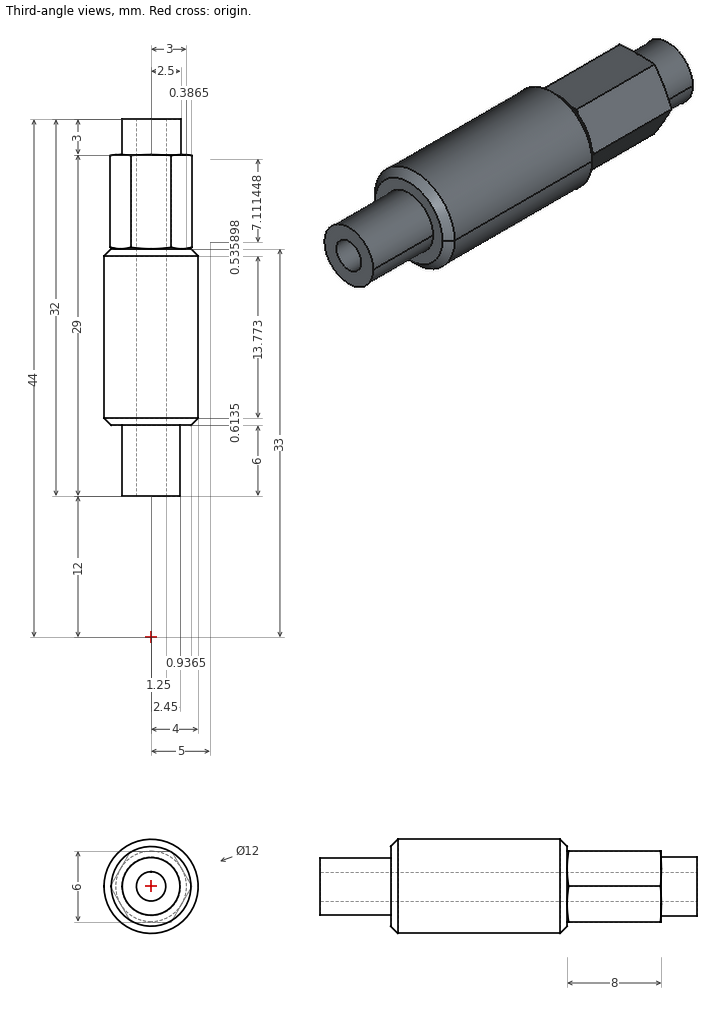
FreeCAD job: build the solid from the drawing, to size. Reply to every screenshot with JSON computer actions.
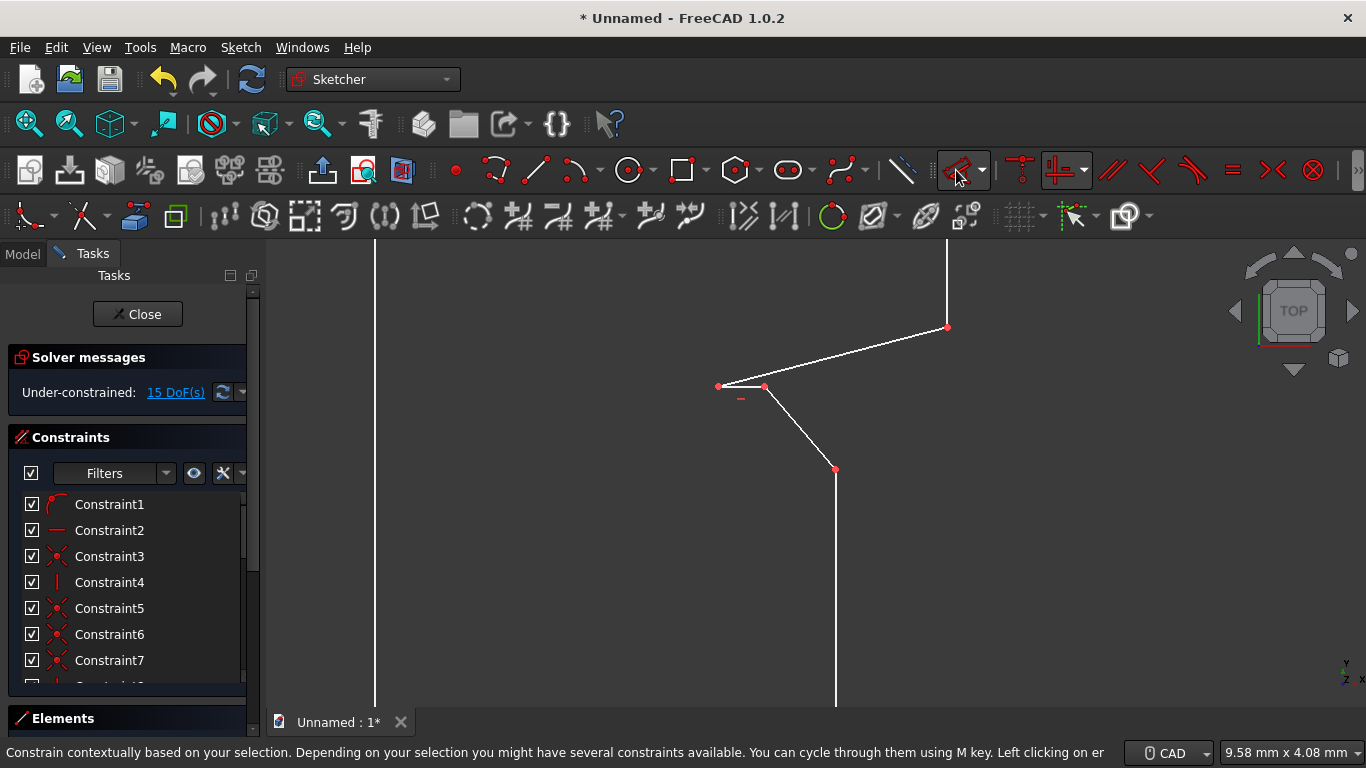
{"action": "scroll", "coordinate": [753, 386], "scroll_direction": "down", "scroll_amount": 14}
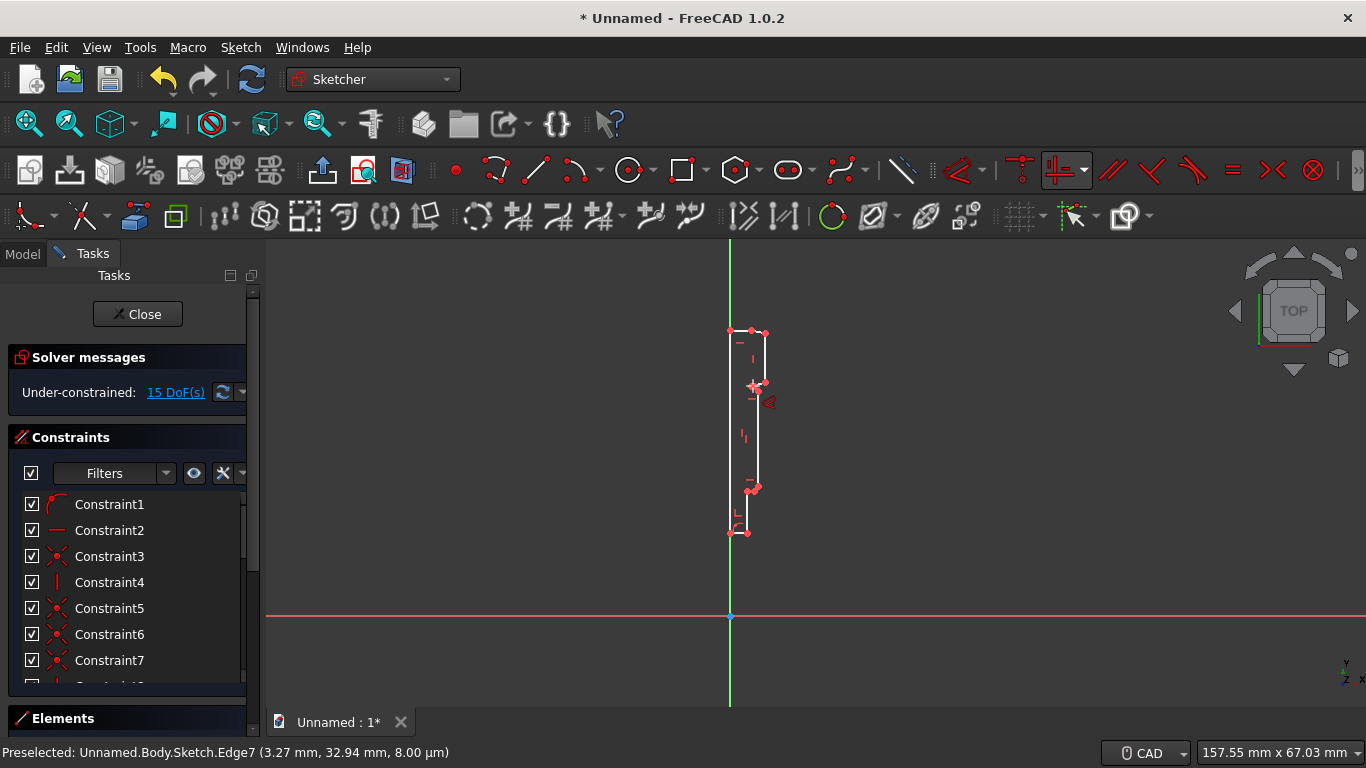
{"action": "left_click", "coordinate": [747, 521]}
{"action": "left_click", "coordinate": [713, 512]}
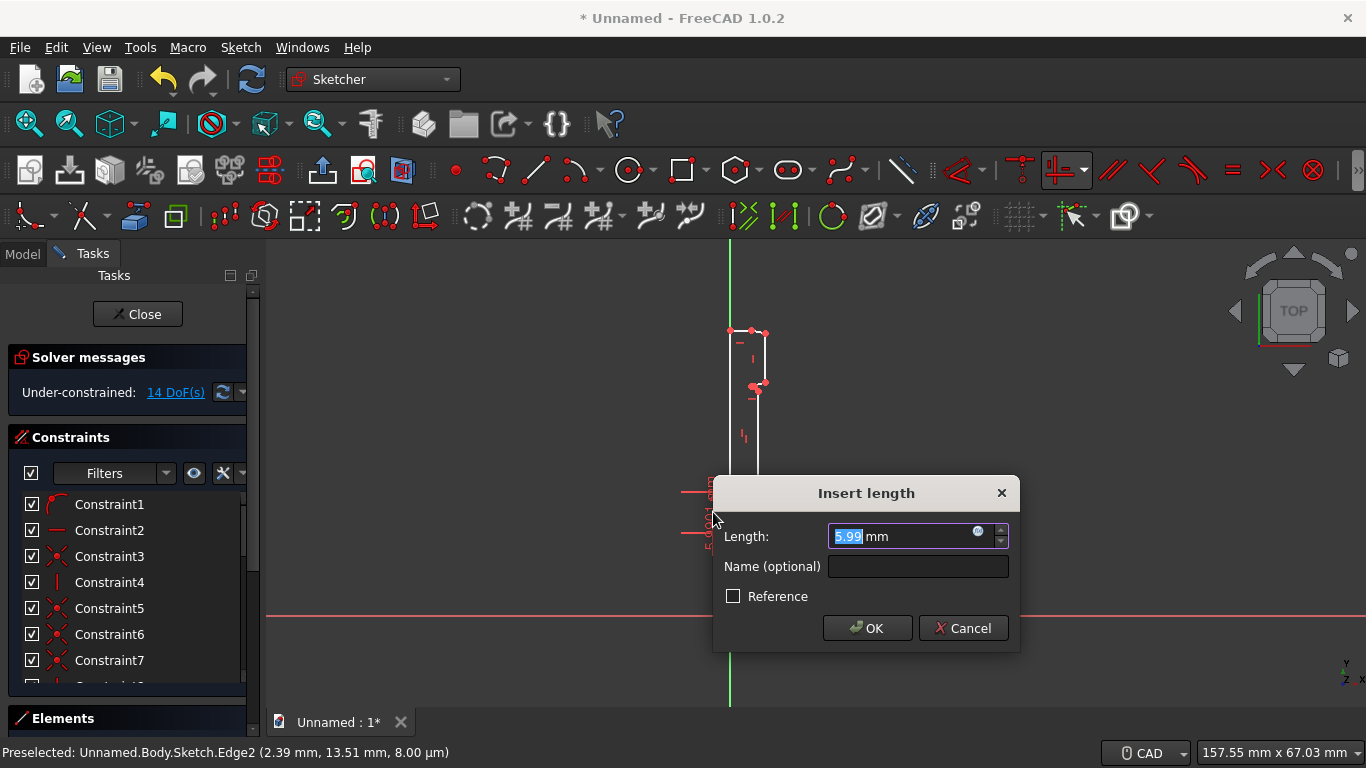
{"action": "type", "text": "6"}
{"action": "key", "text": "Return"}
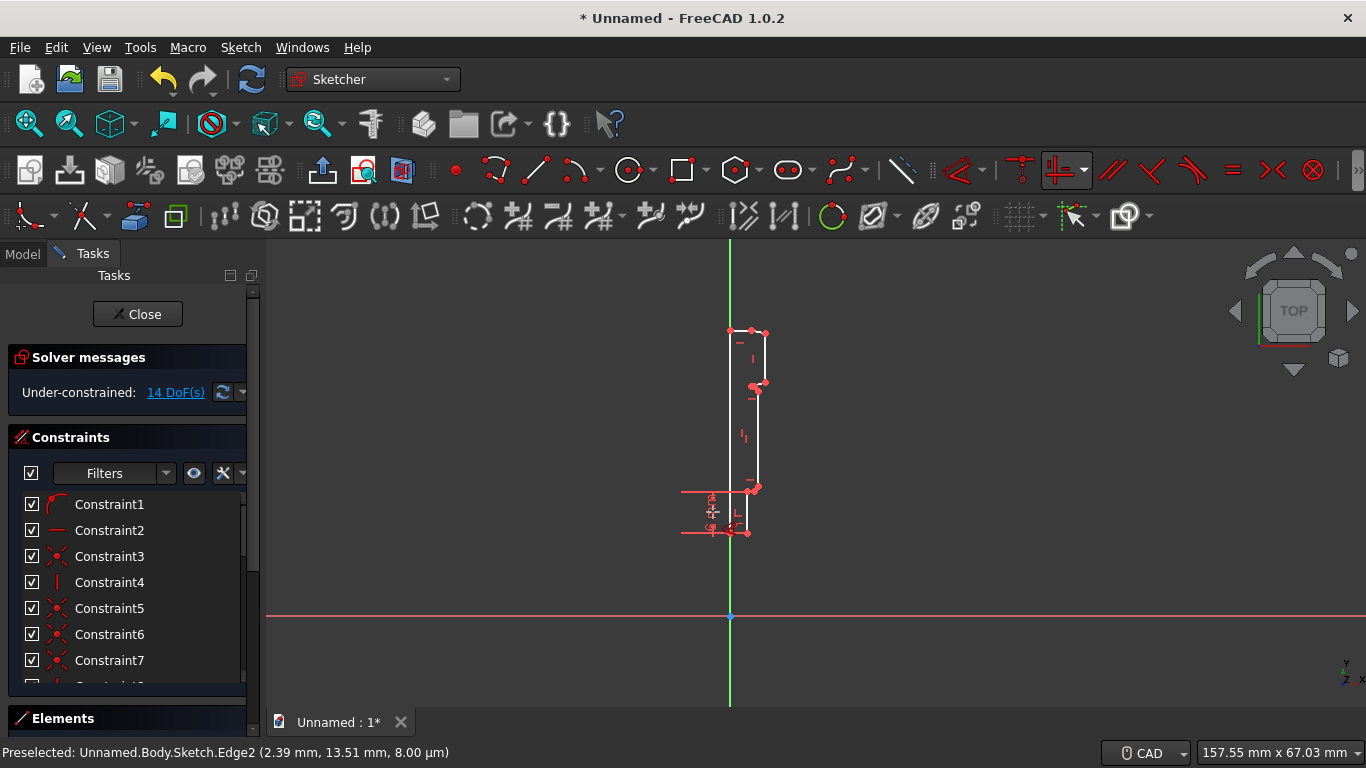
{"action": "scroll", "coordinate": [741, 331], "scroll_direction": "up", "scroll_amount": 4}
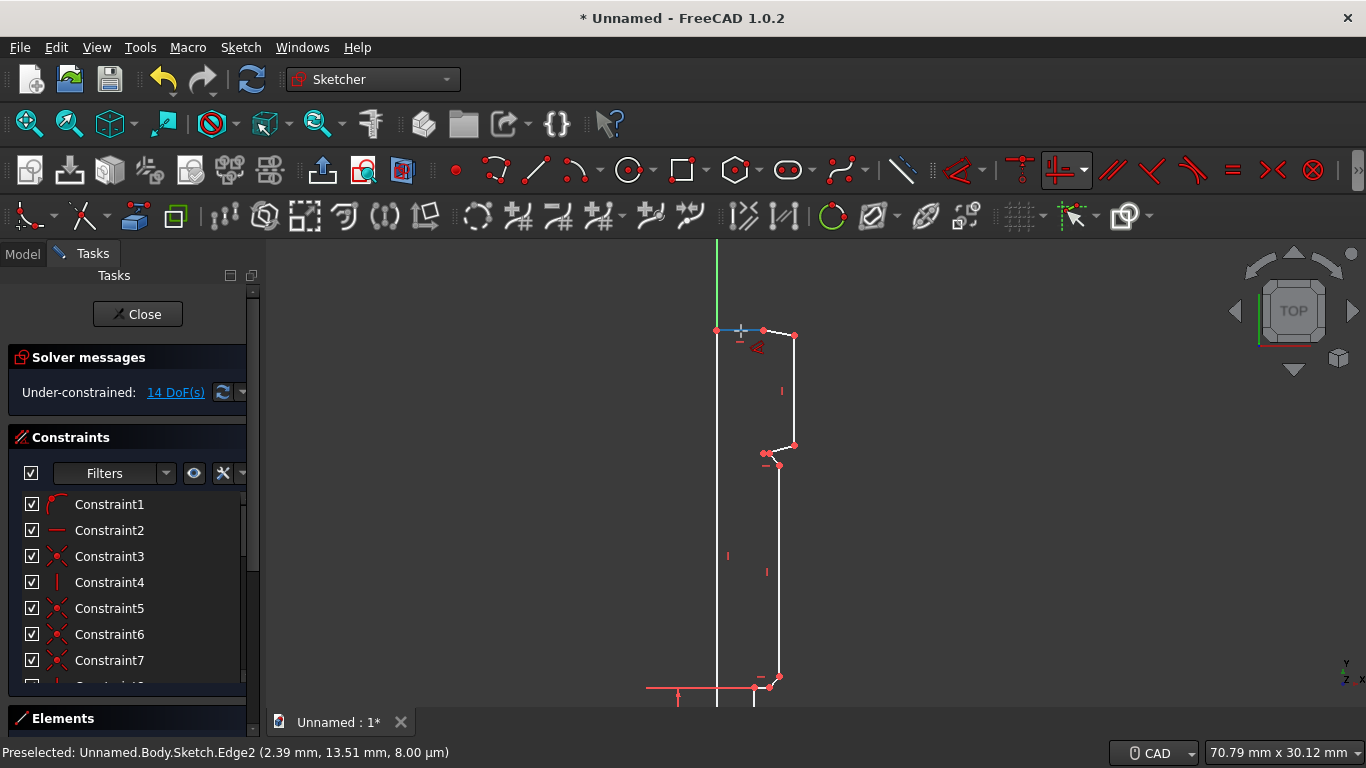
{"action": "left_click", "coordinate": [740, 330]}
{"action": "left_click", "coordinate": [740, 296]}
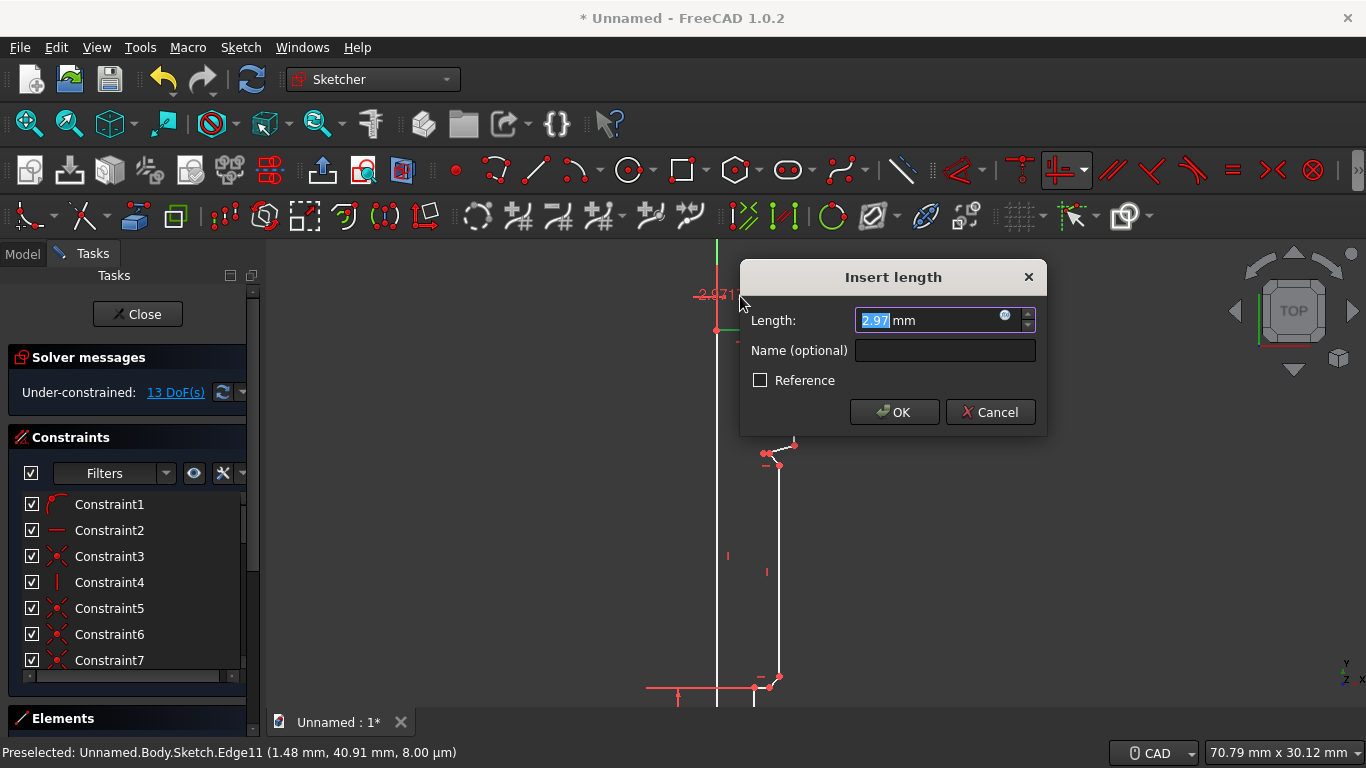
{"action": "type", "text": "3"}
{"action": "key", "text": "Return"}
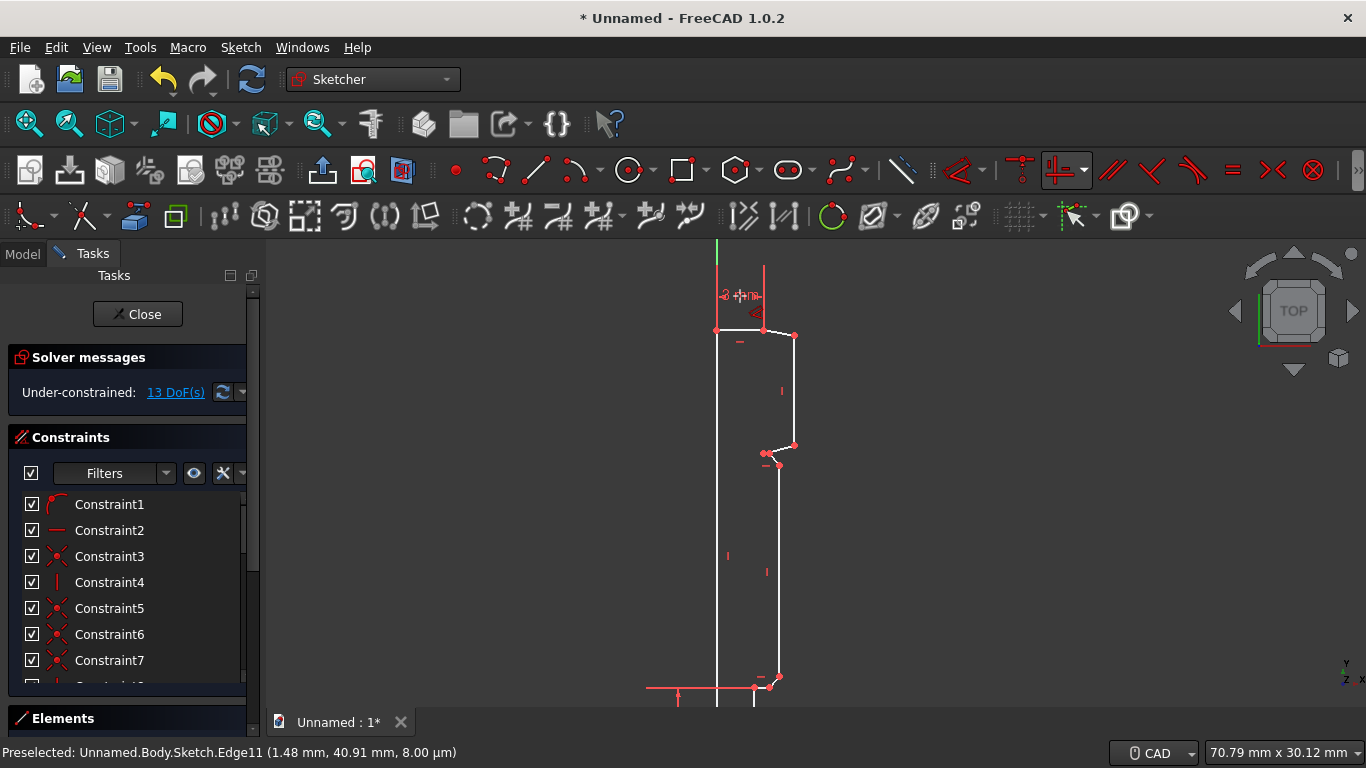
{"action": "left_click", "coordinate": [717, 465]}
{"action": "left_click", "coordinate": [683, 505]}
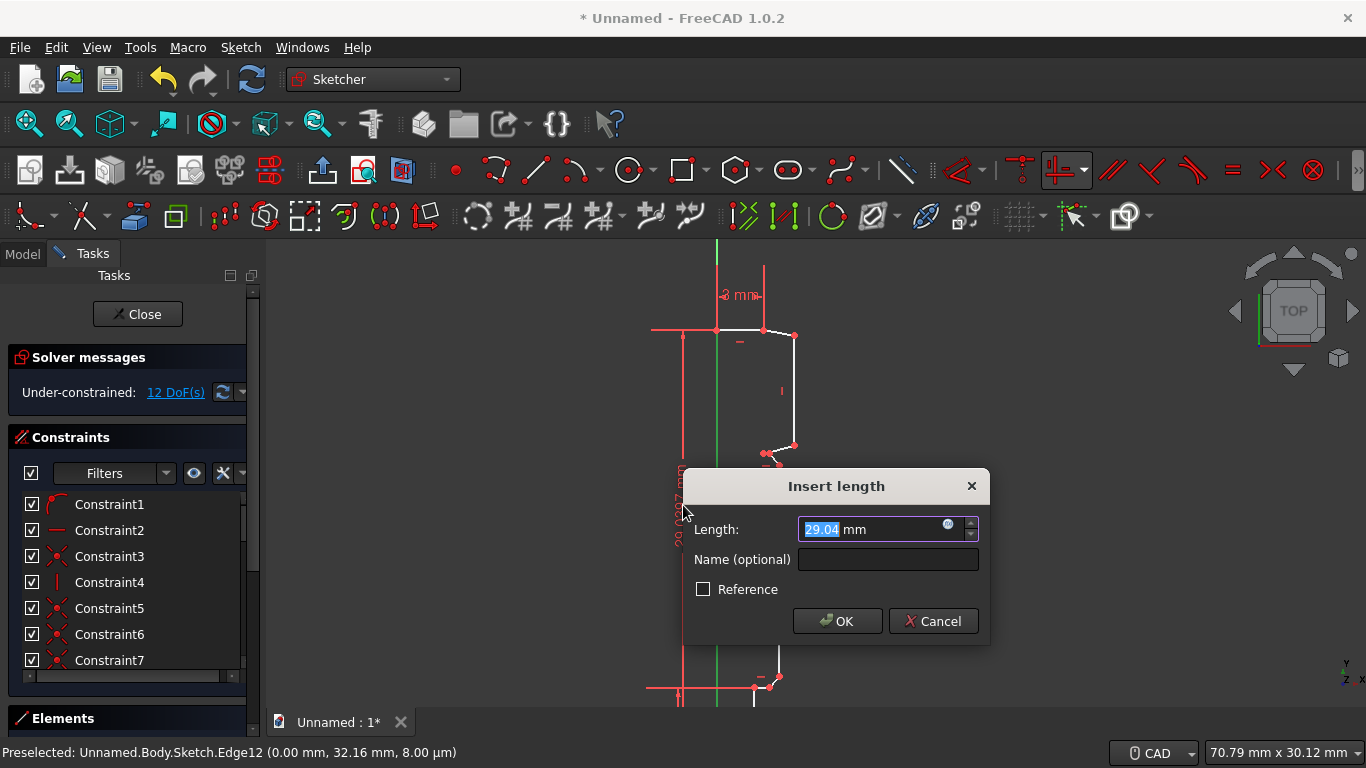
{"action": "type", "text": "29"}
{"action": "key", "text": "Return"}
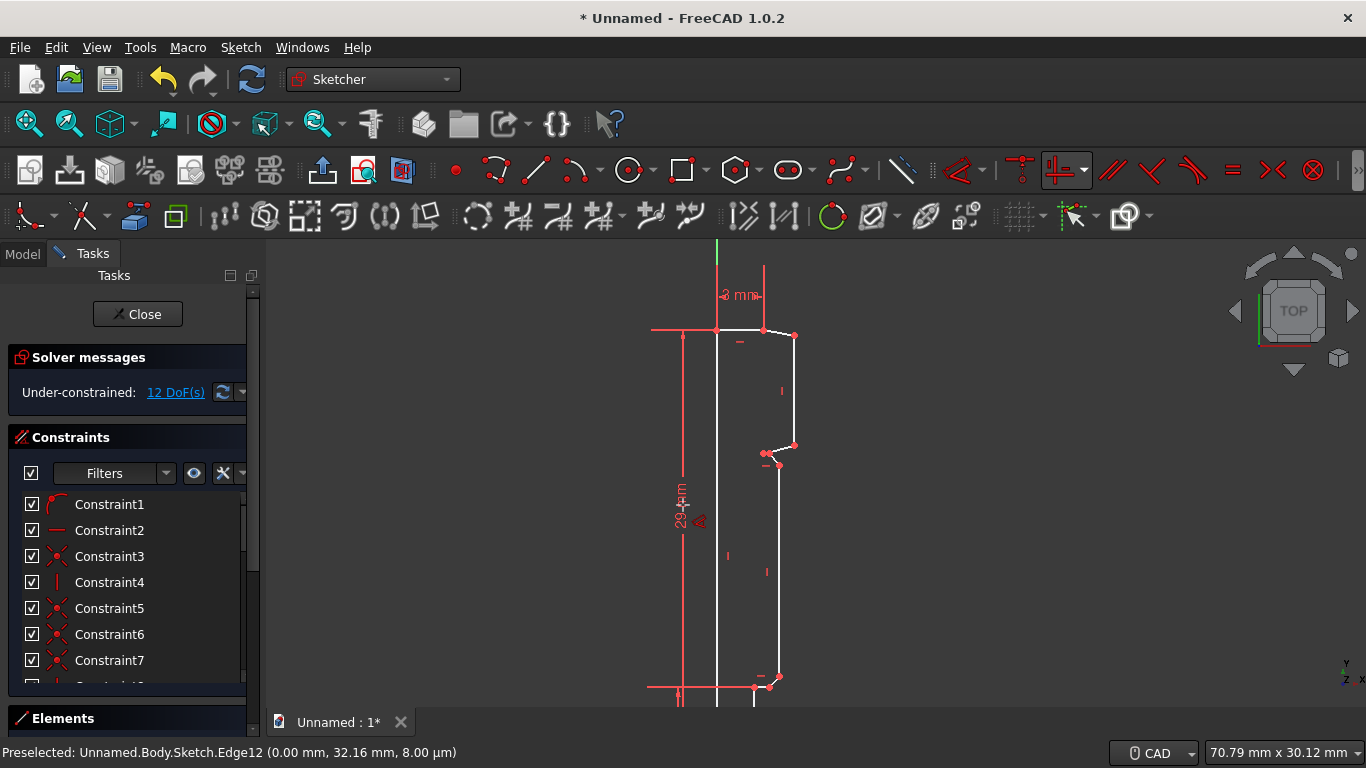
{"action": "left_click", "coordinate": [779, 677]}
{"action": "left_click", "coordinate": [748, 643]}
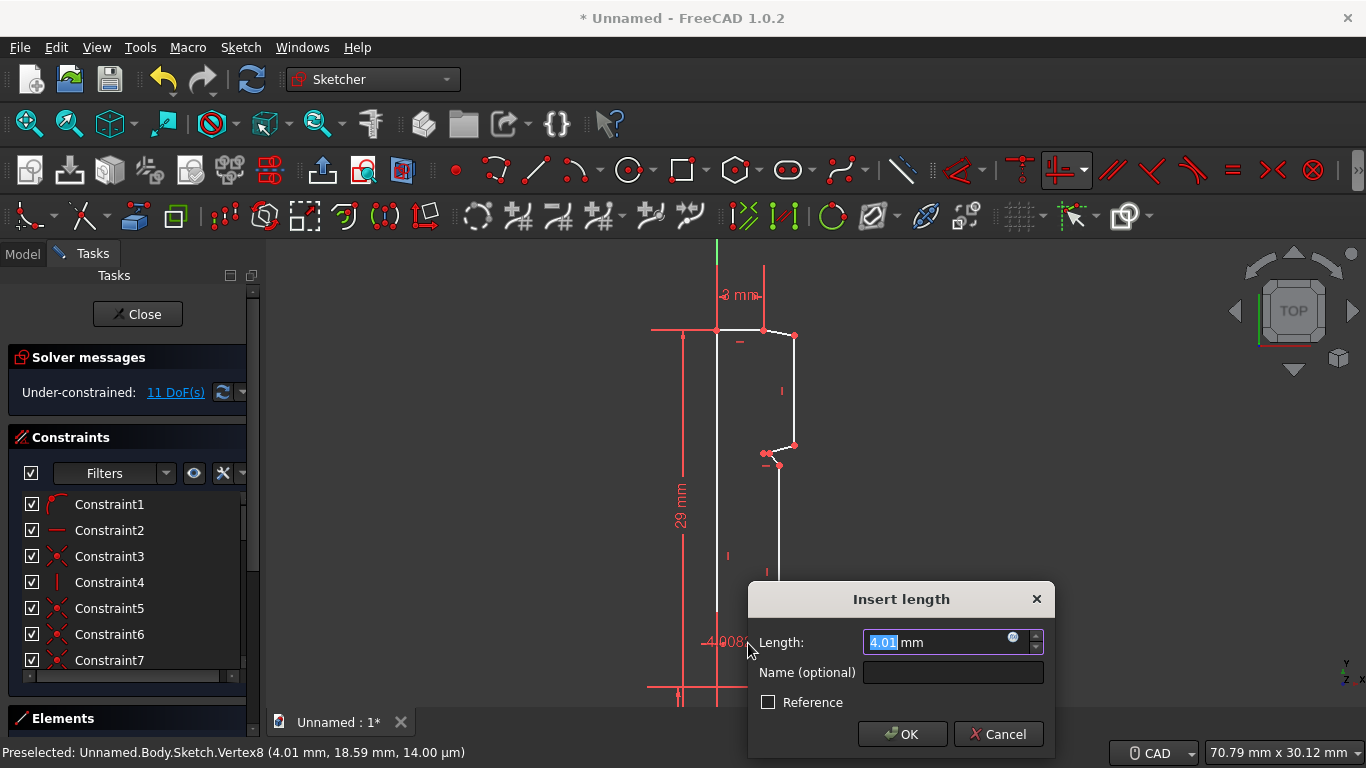
{"action": "type", "text": "4"}
{"action": "key", "text": "Return"}